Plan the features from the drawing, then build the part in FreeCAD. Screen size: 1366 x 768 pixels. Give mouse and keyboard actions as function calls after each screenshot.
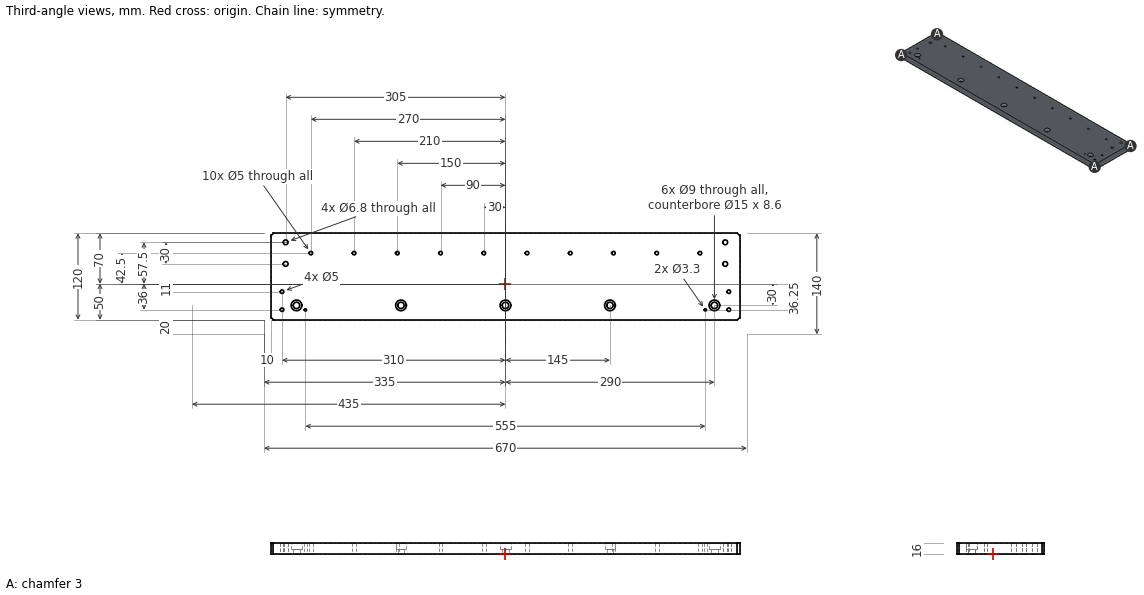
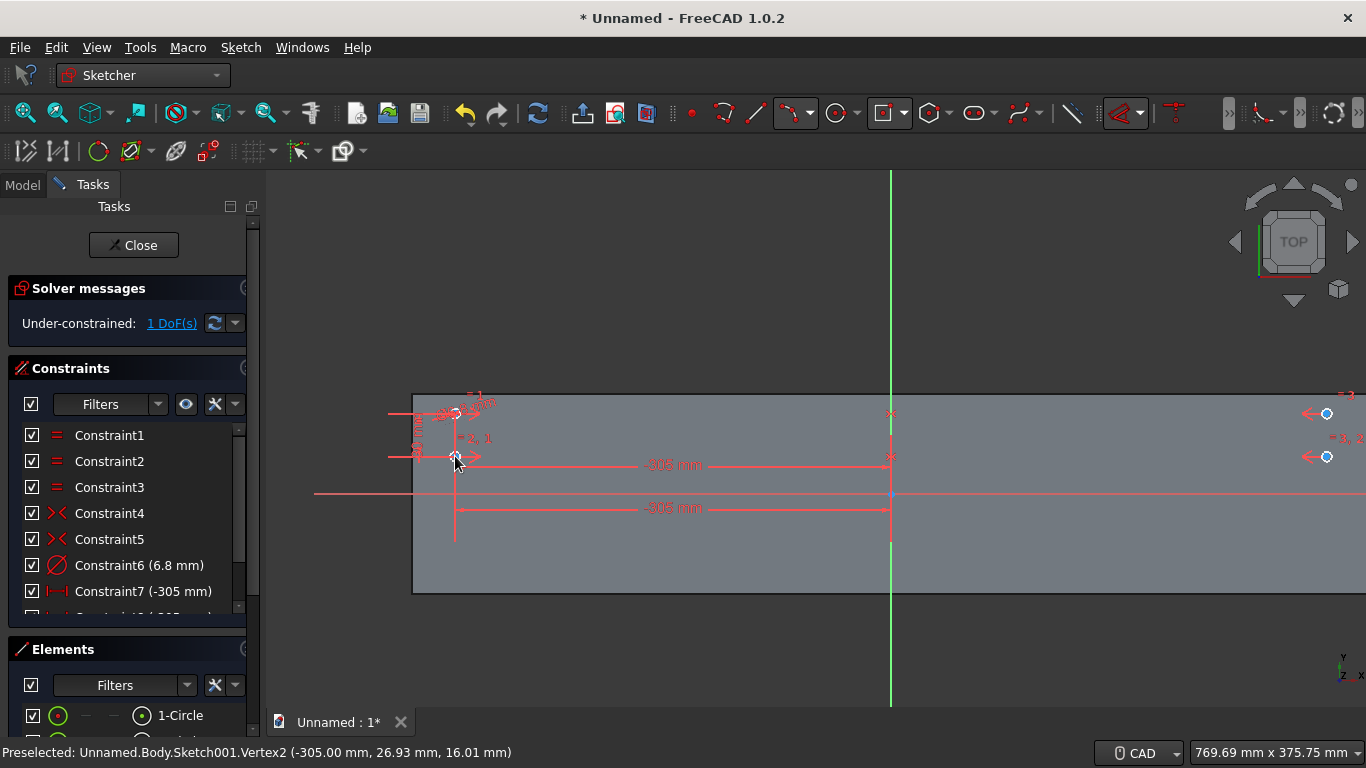
click(455, 414)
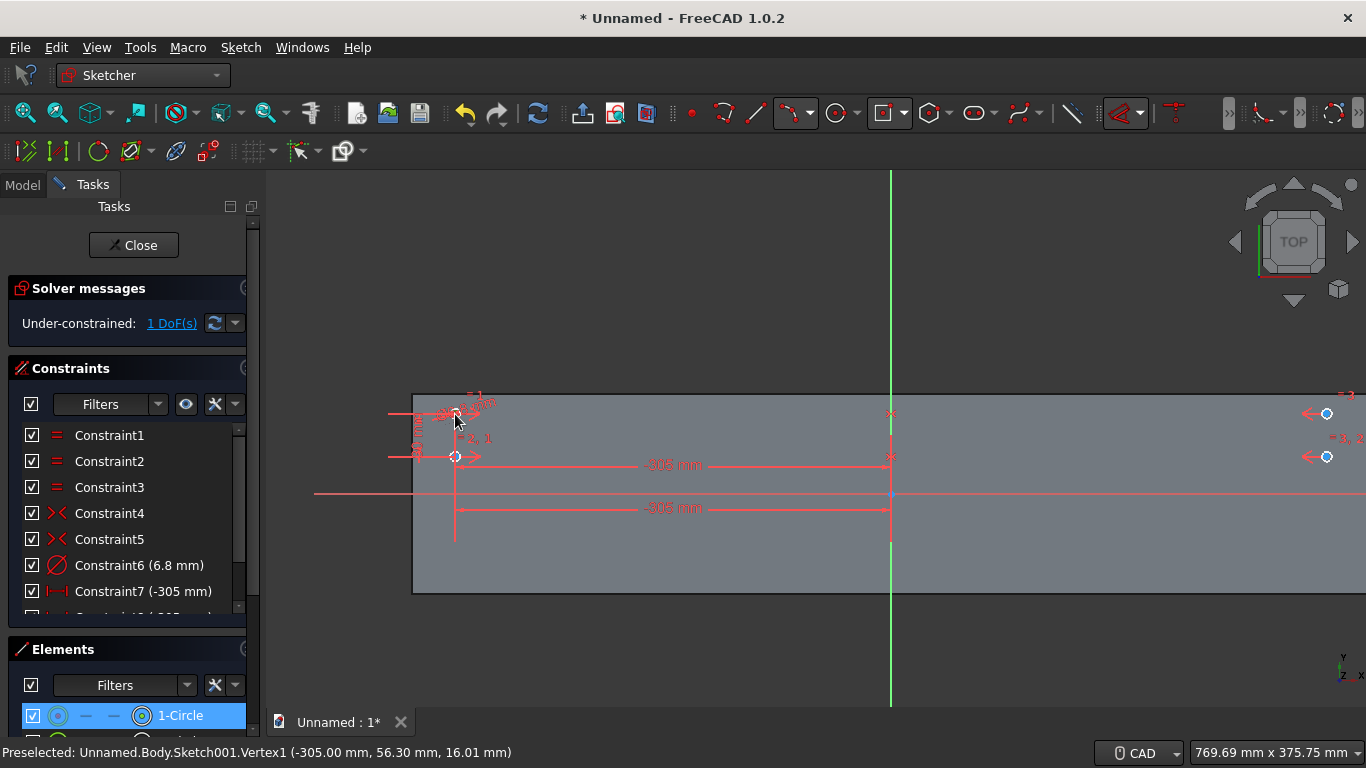
key(i)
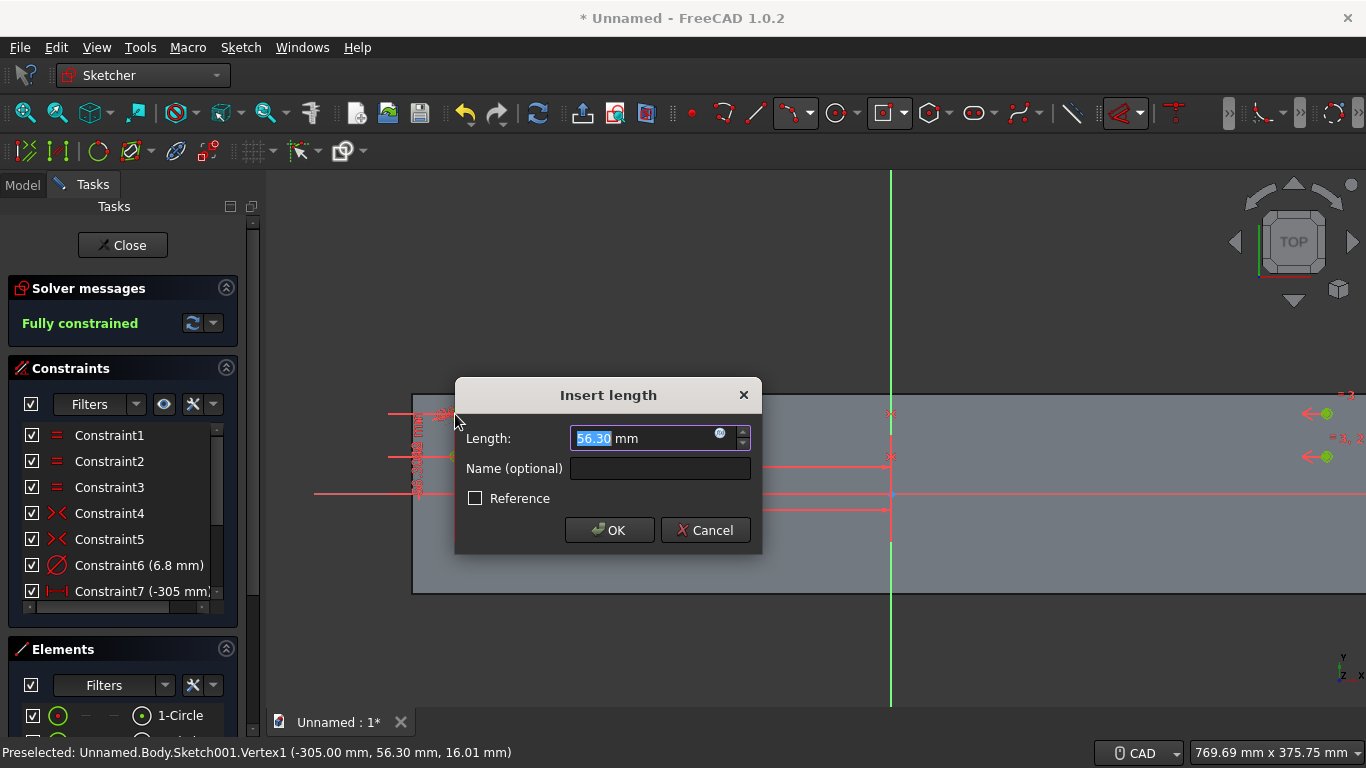
text(57.5)
key(Return)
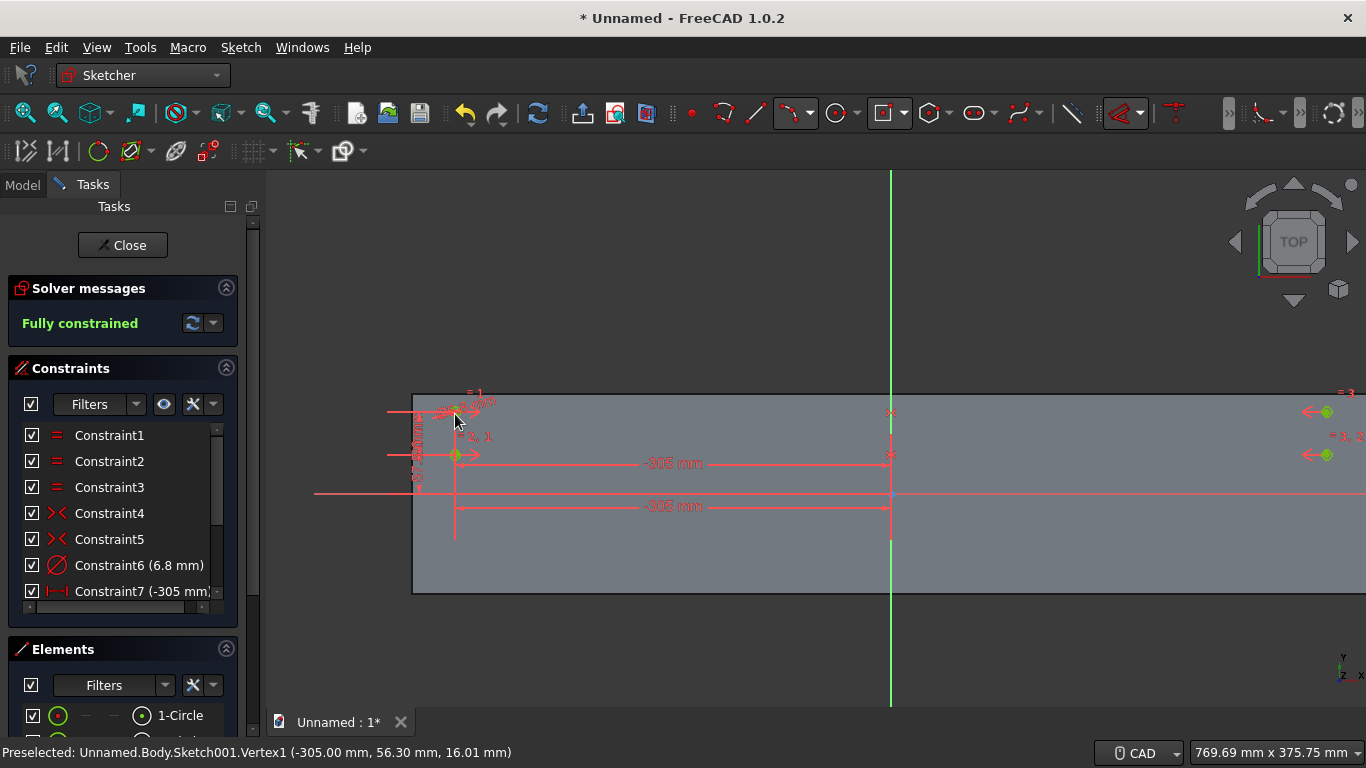
click(123, 245)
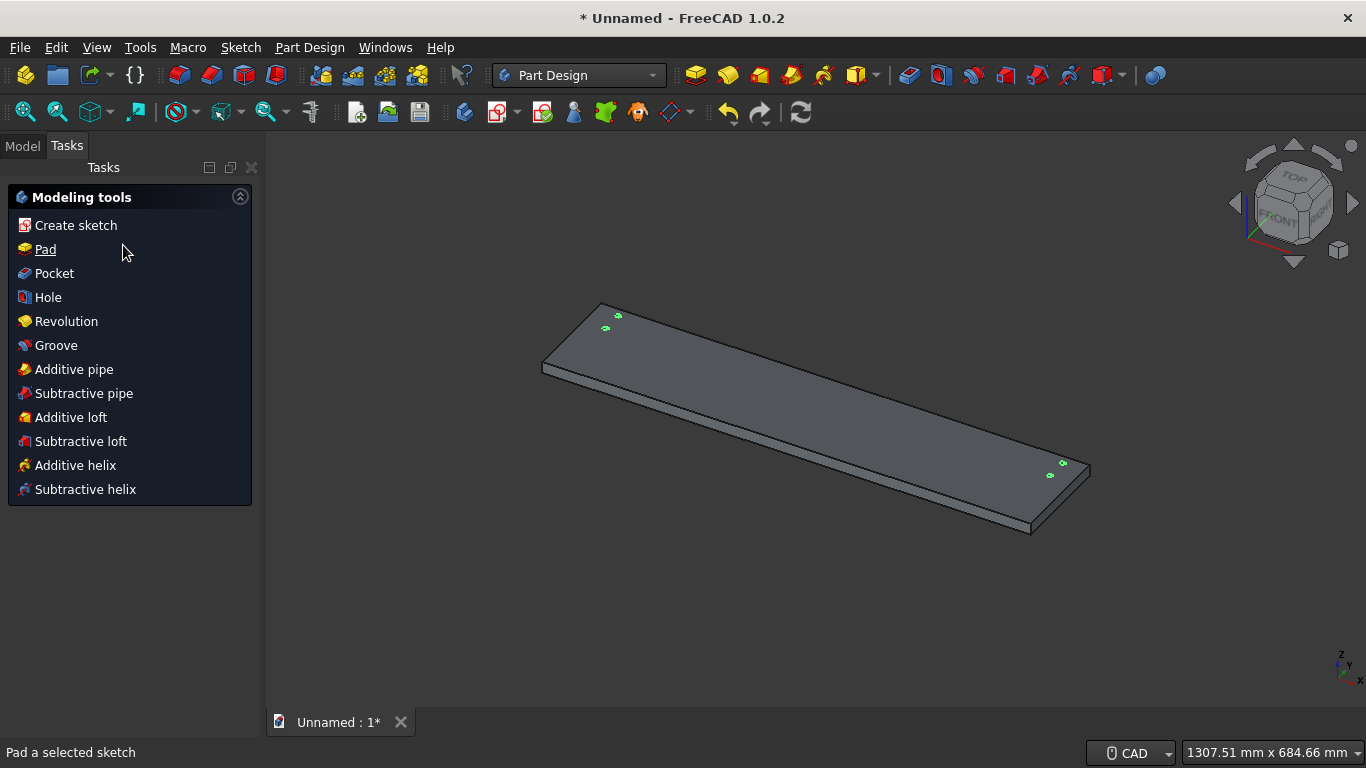
click(942, 76)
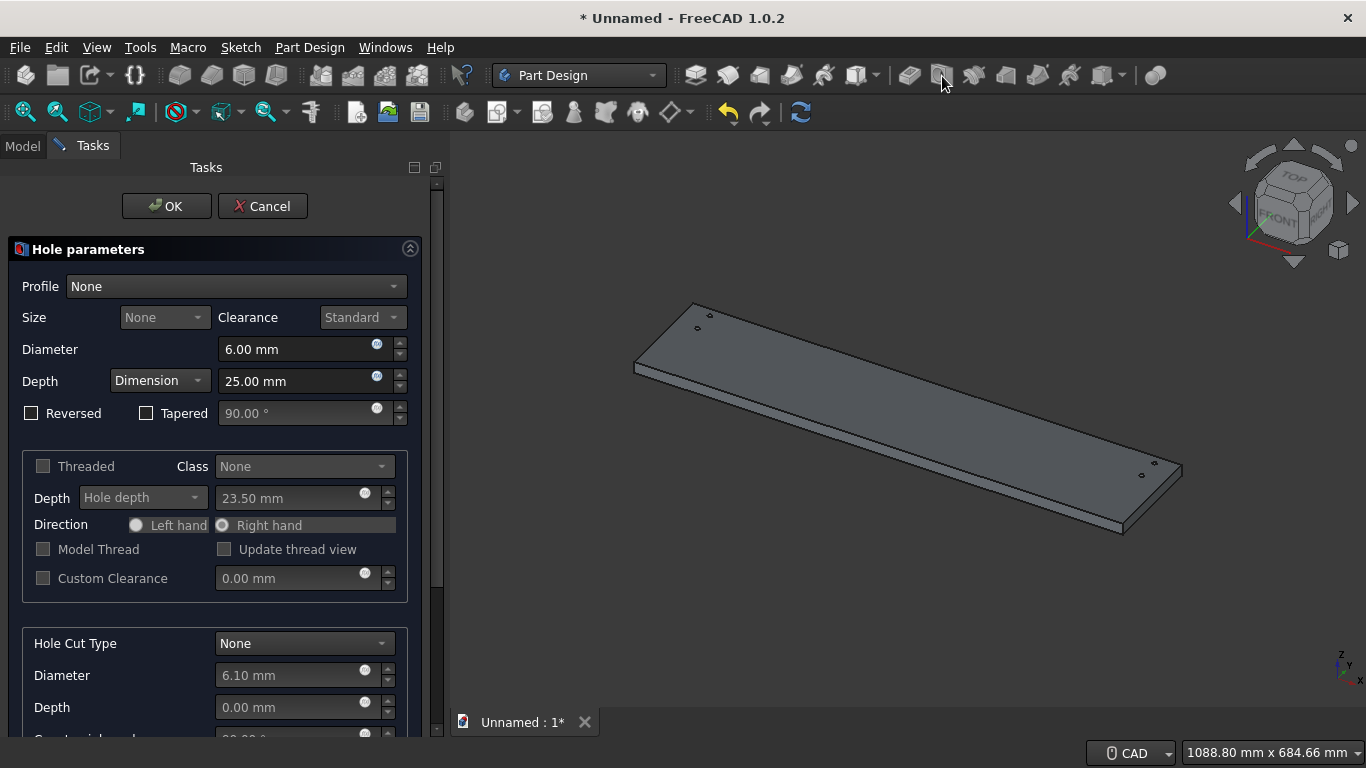
triple_click(305, 349)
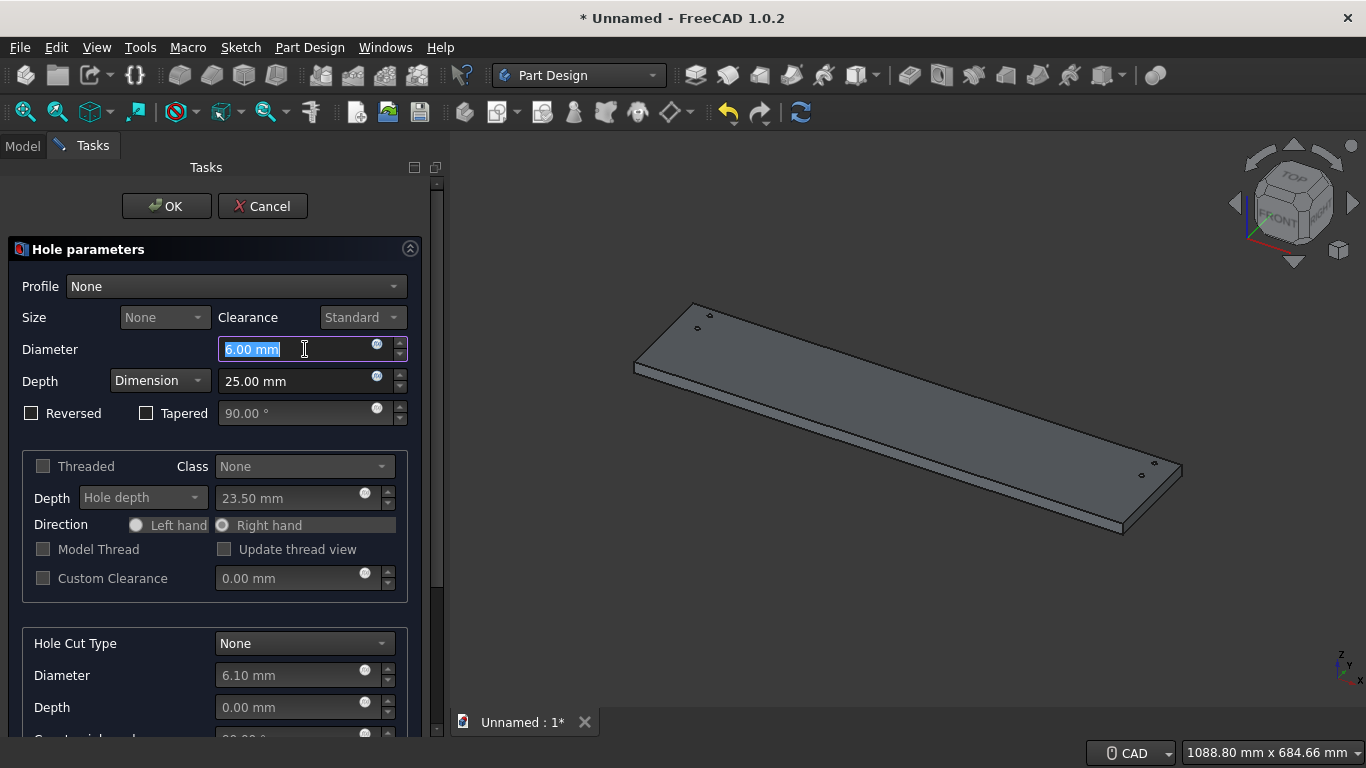
text(6.8)
key(Tab)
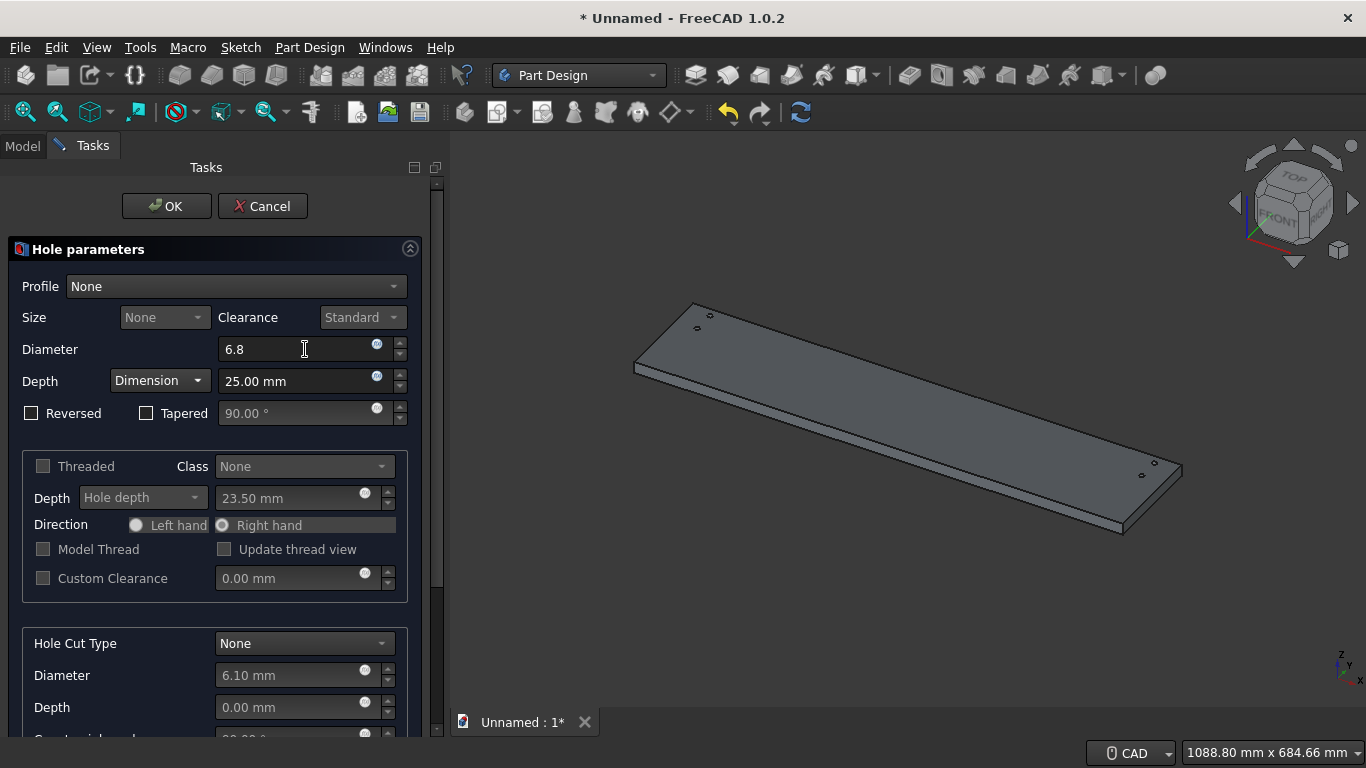
click(161, 380)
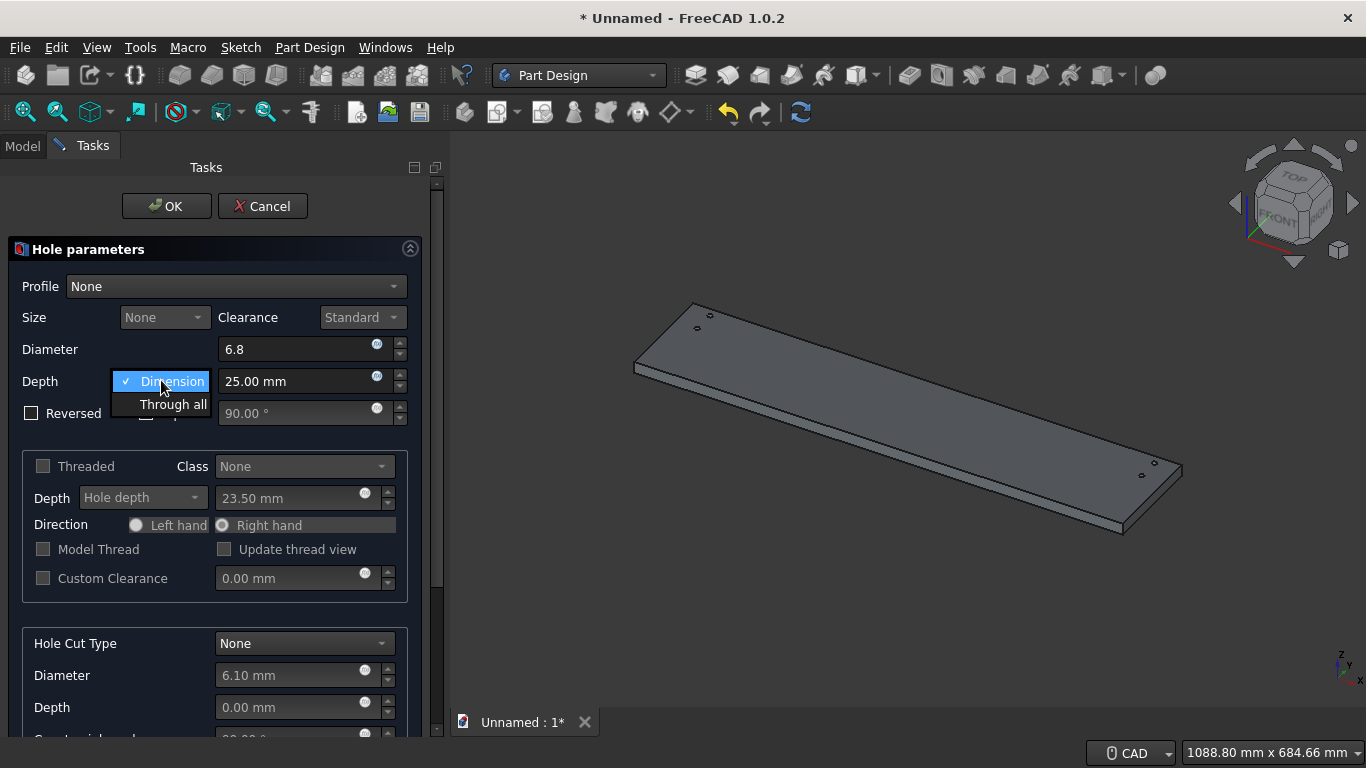
click(160, 404)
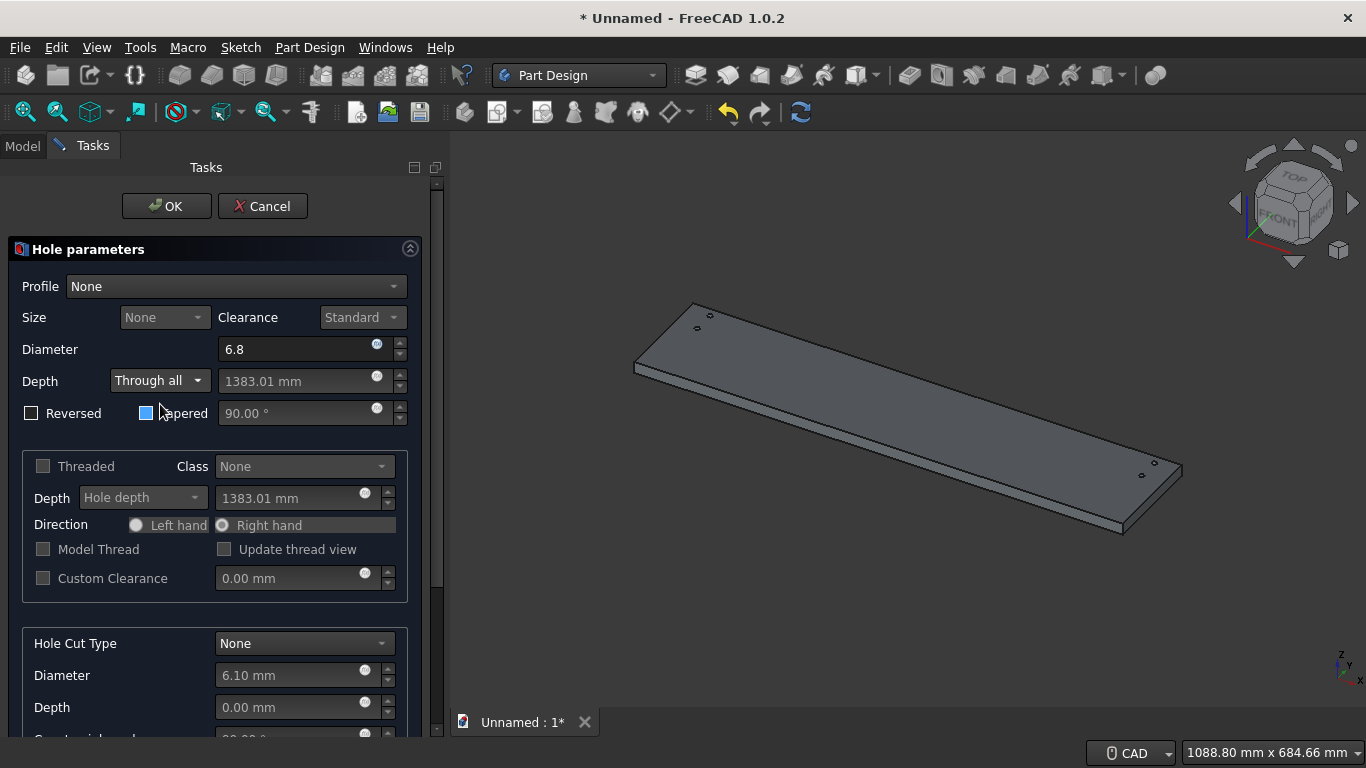
click(167, 206)